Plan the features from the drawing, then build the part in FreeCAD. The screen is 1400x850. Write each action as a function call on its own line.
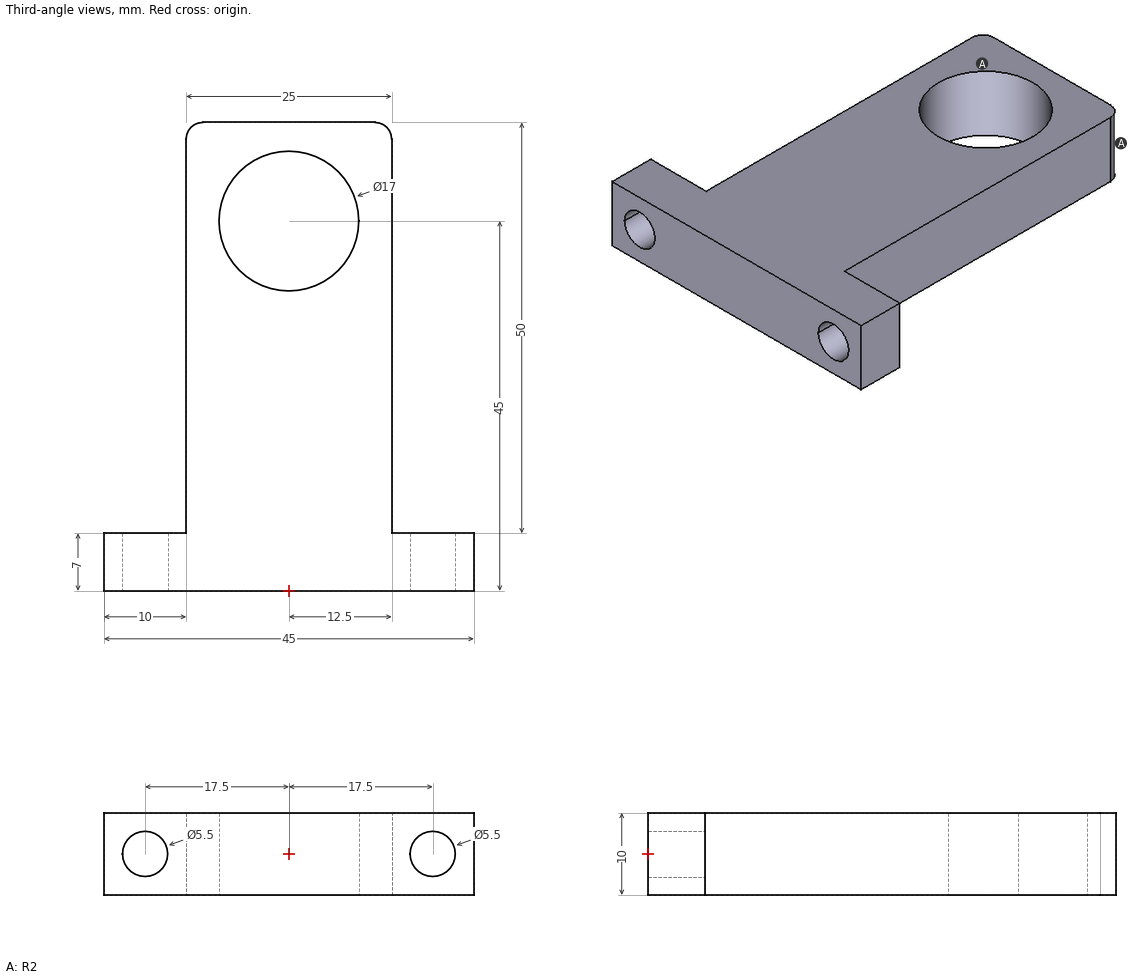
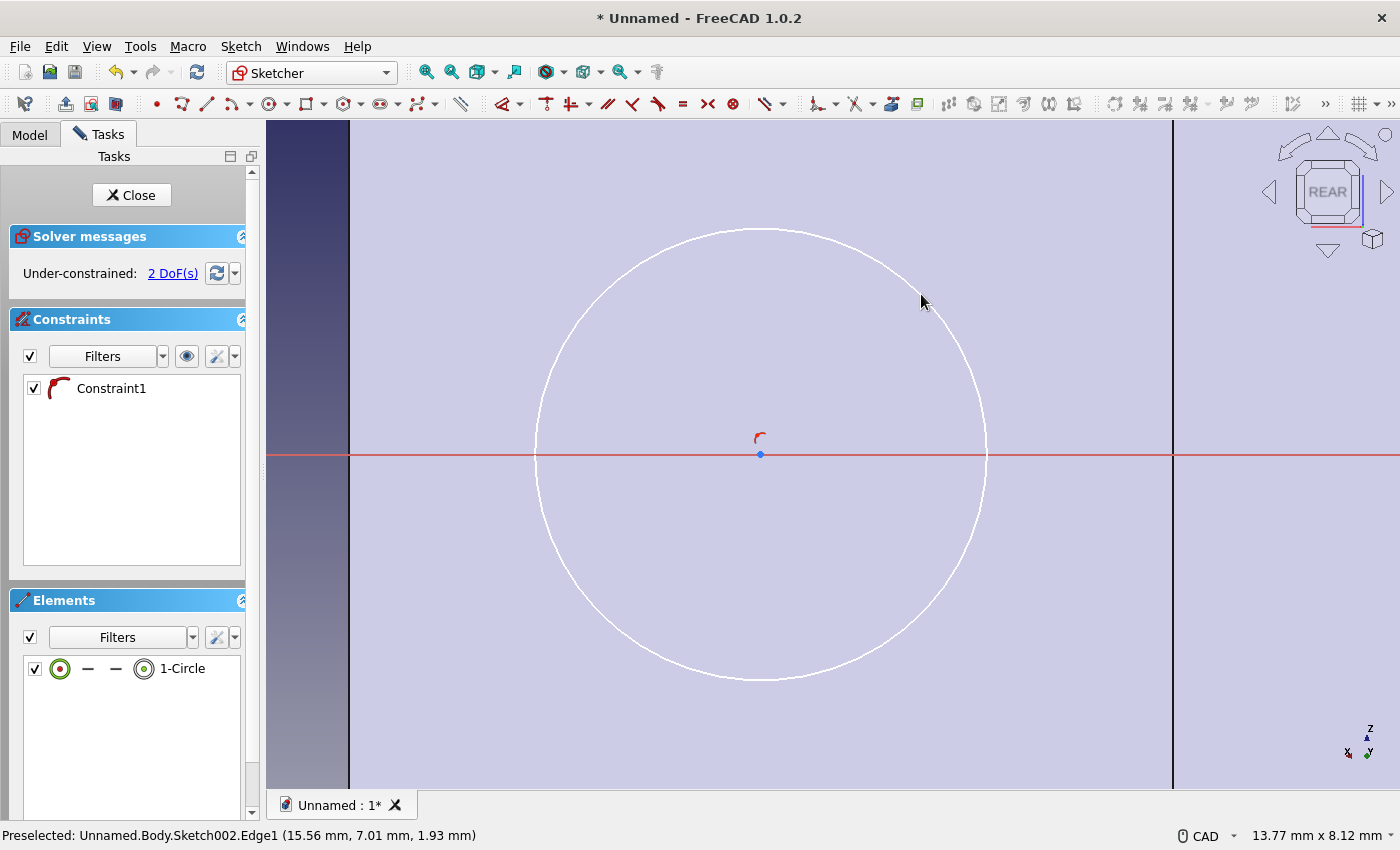
click(502, 104)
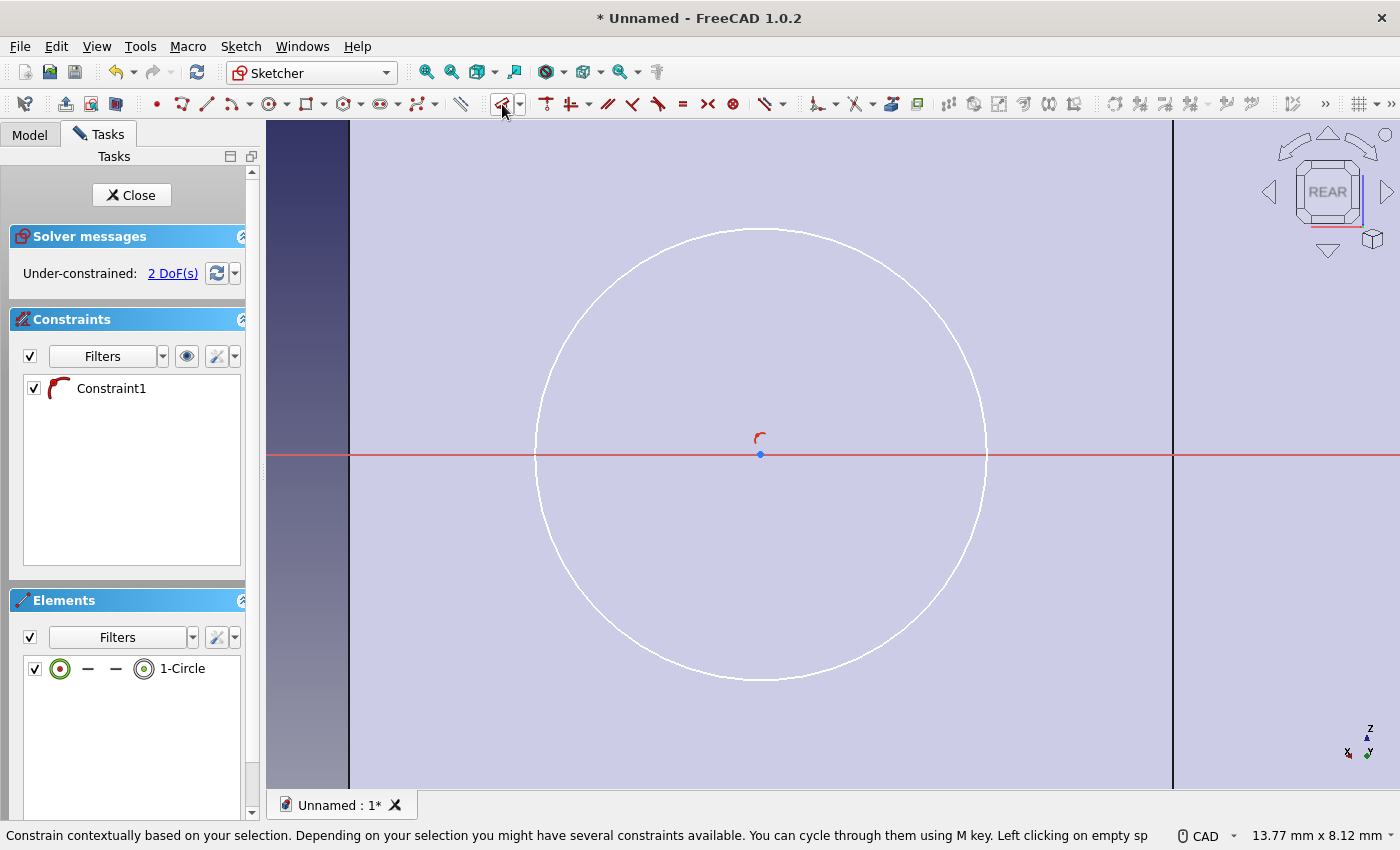
click(920, 294)
click(943, 271)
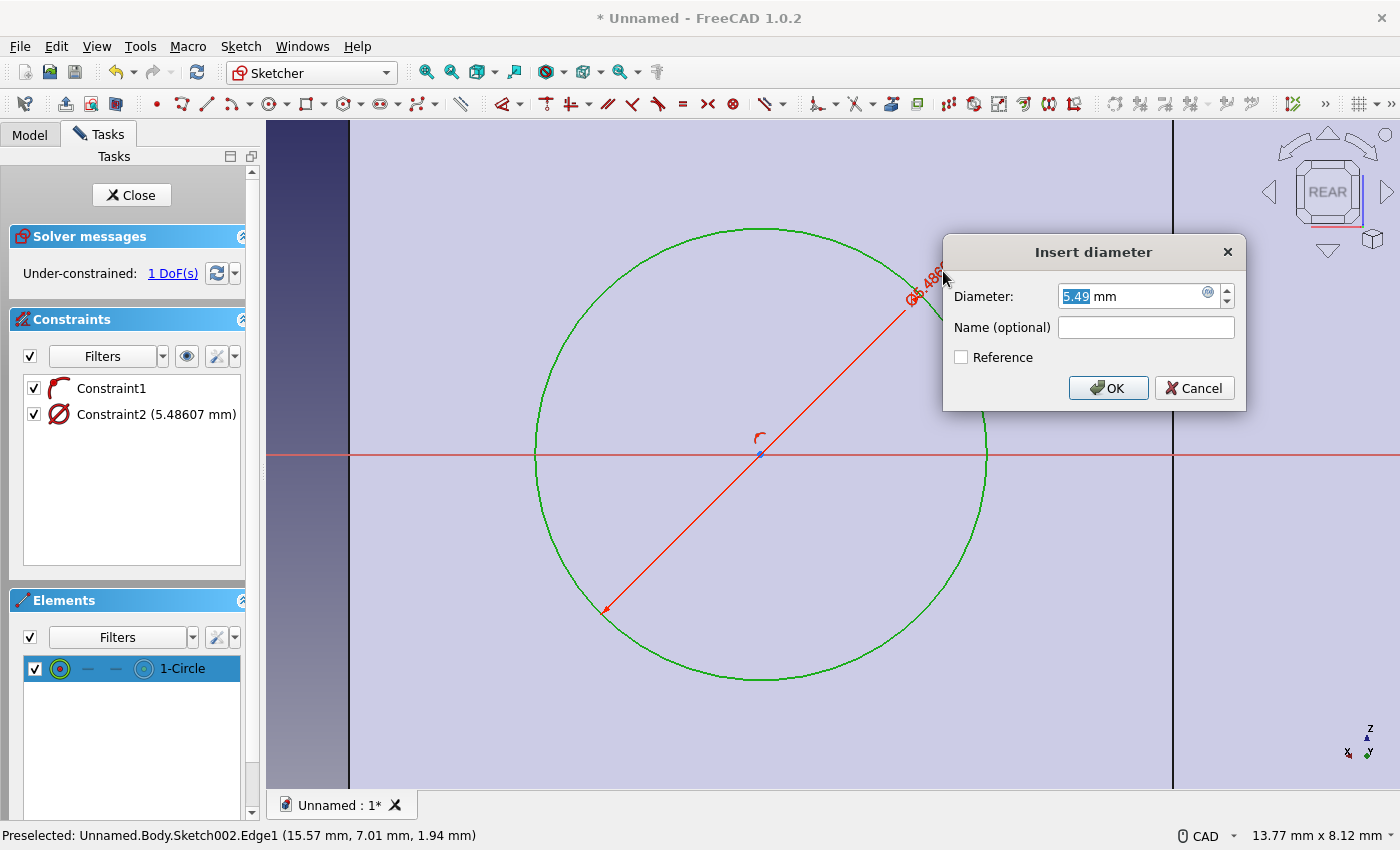
text(5.5)
key(Return)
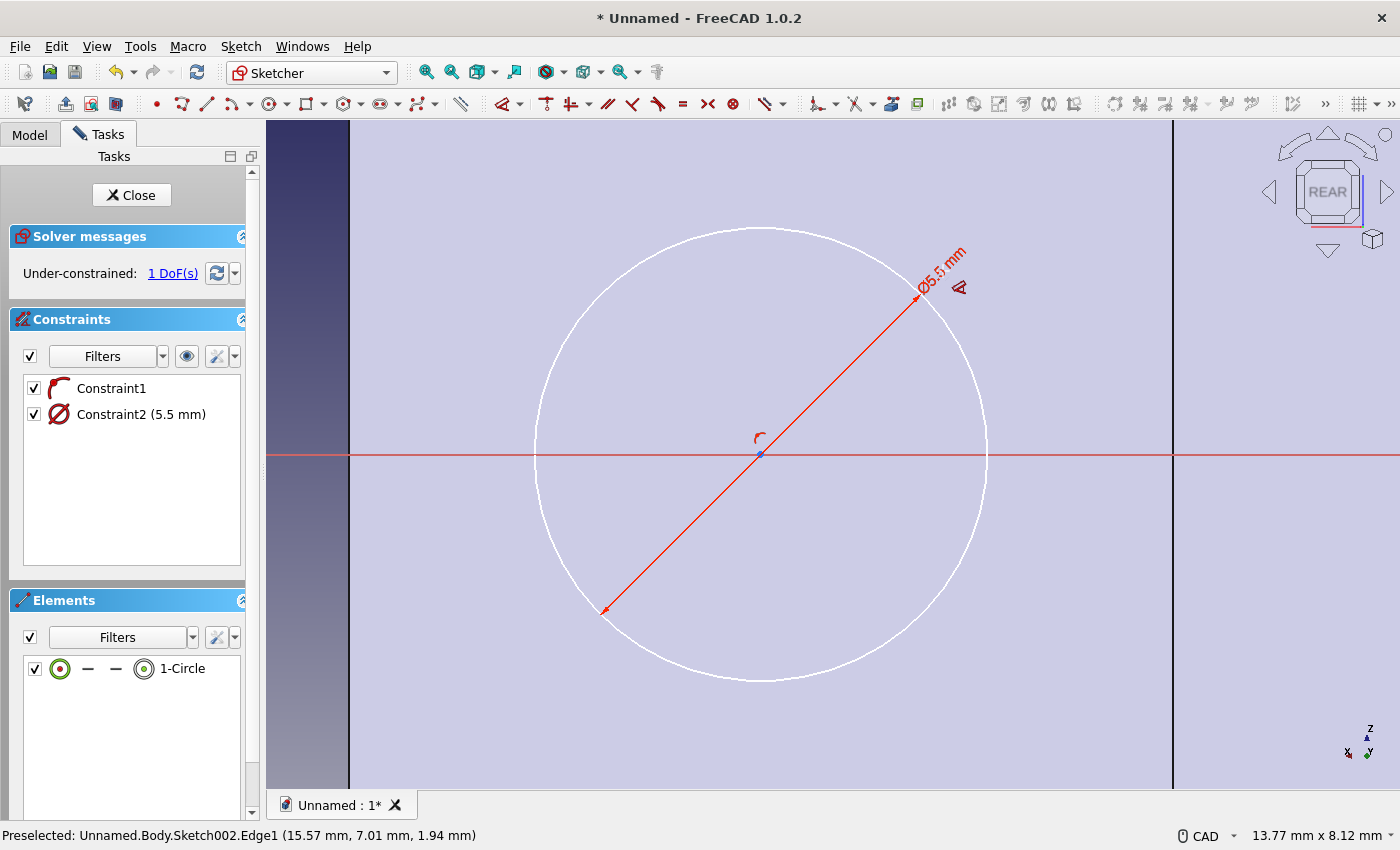
click(761, 454)
click(889, 488)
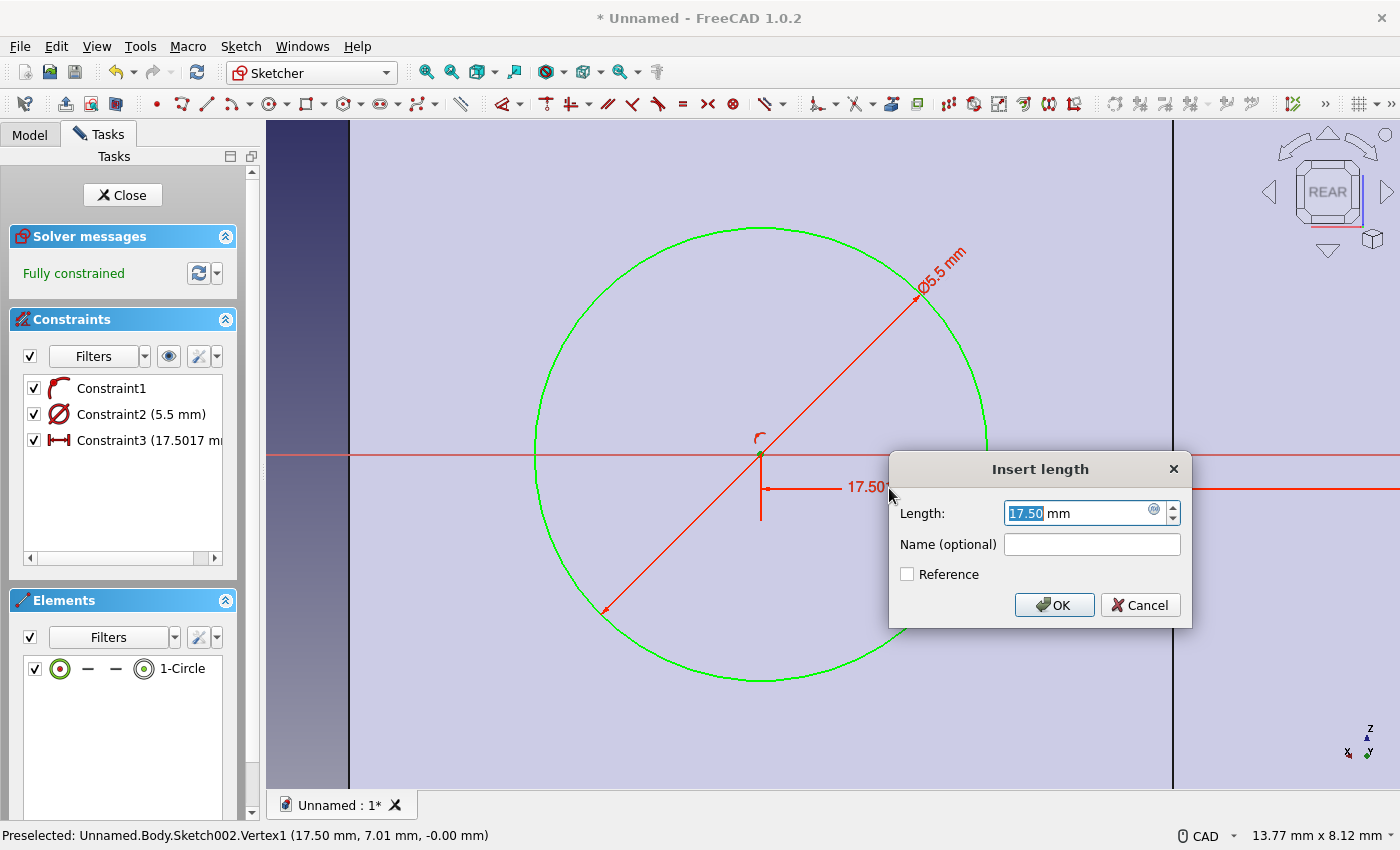
text(17.5)
key(Return)
key(Escape)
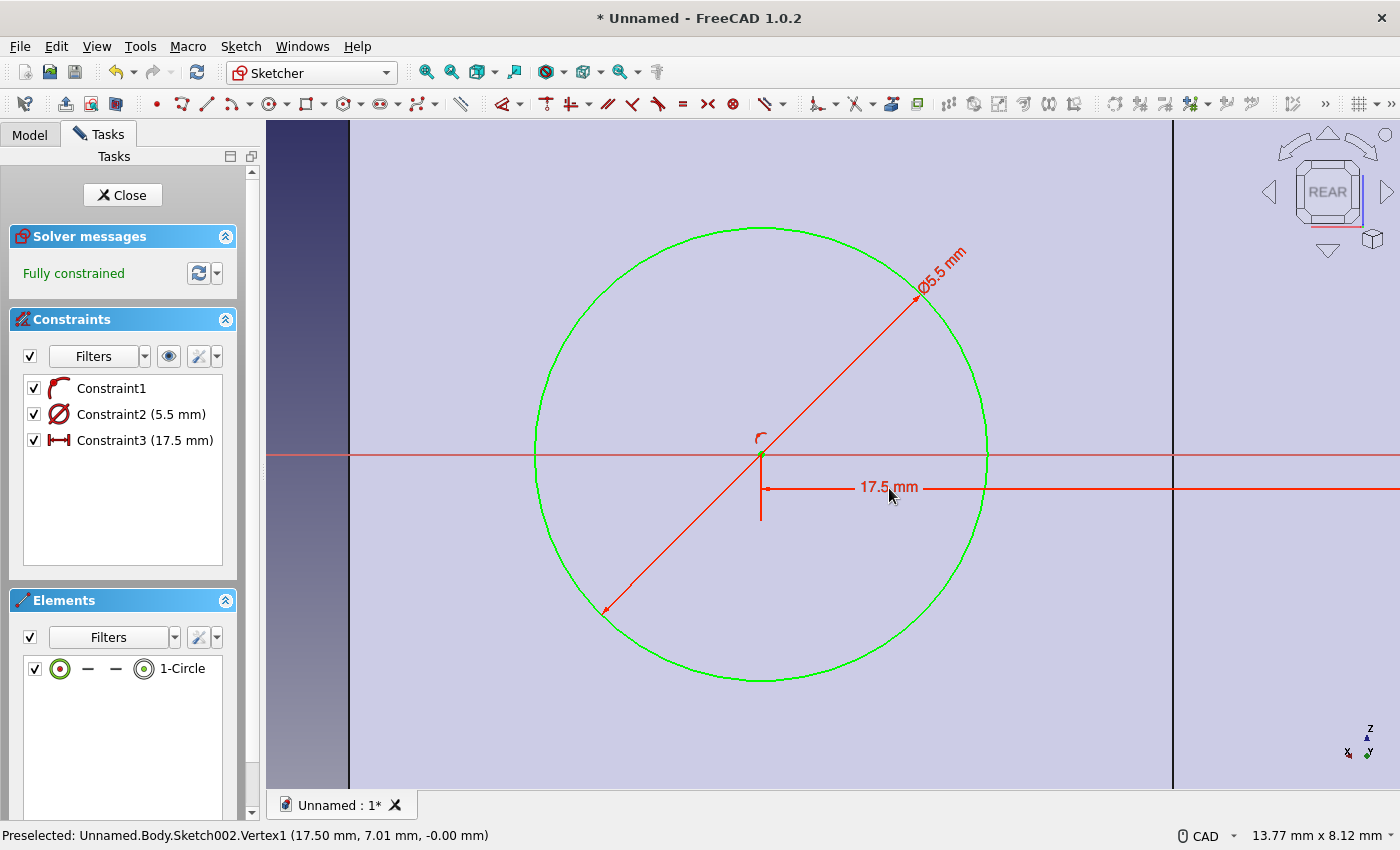
click(123, 195)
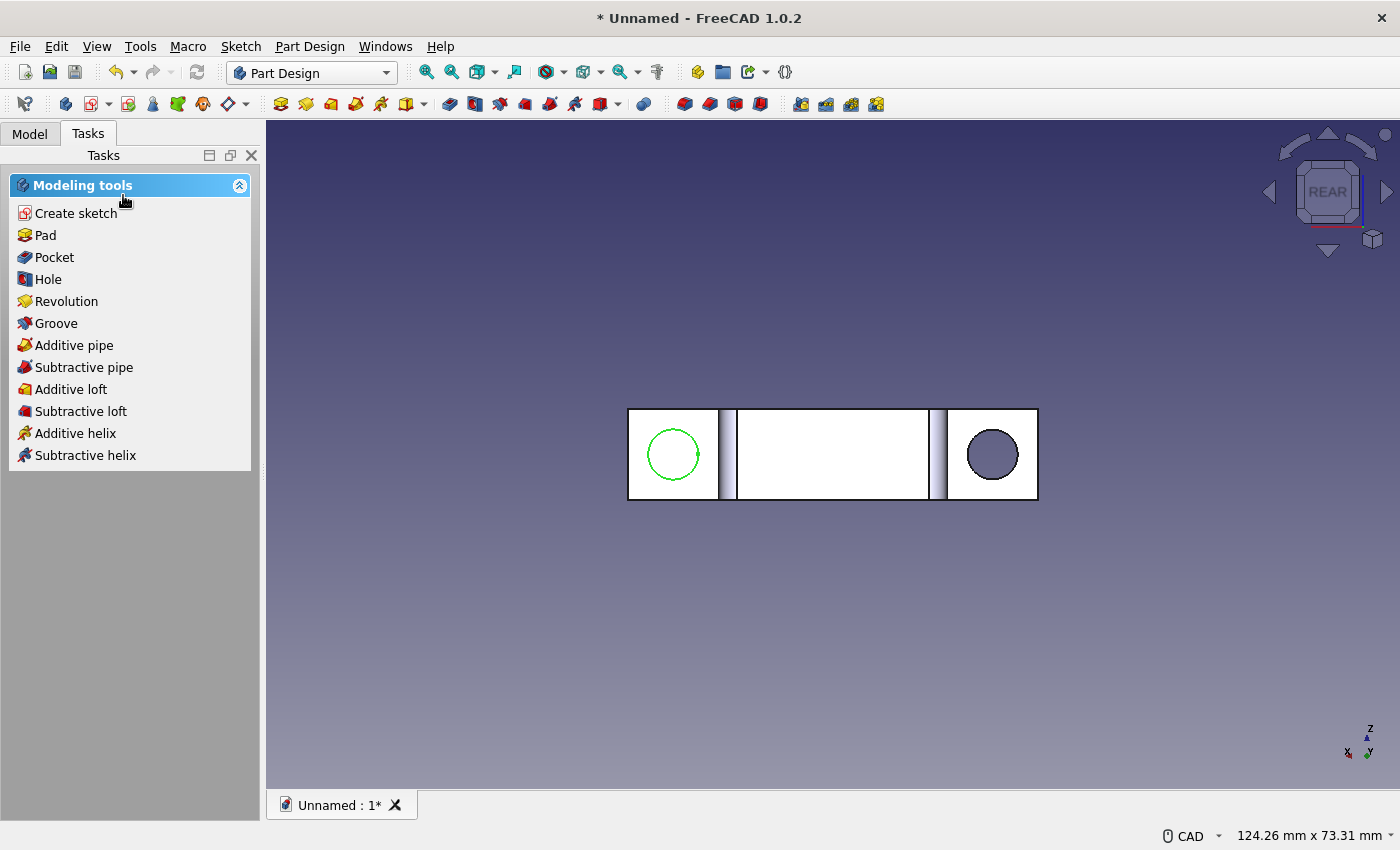
click(450, 104)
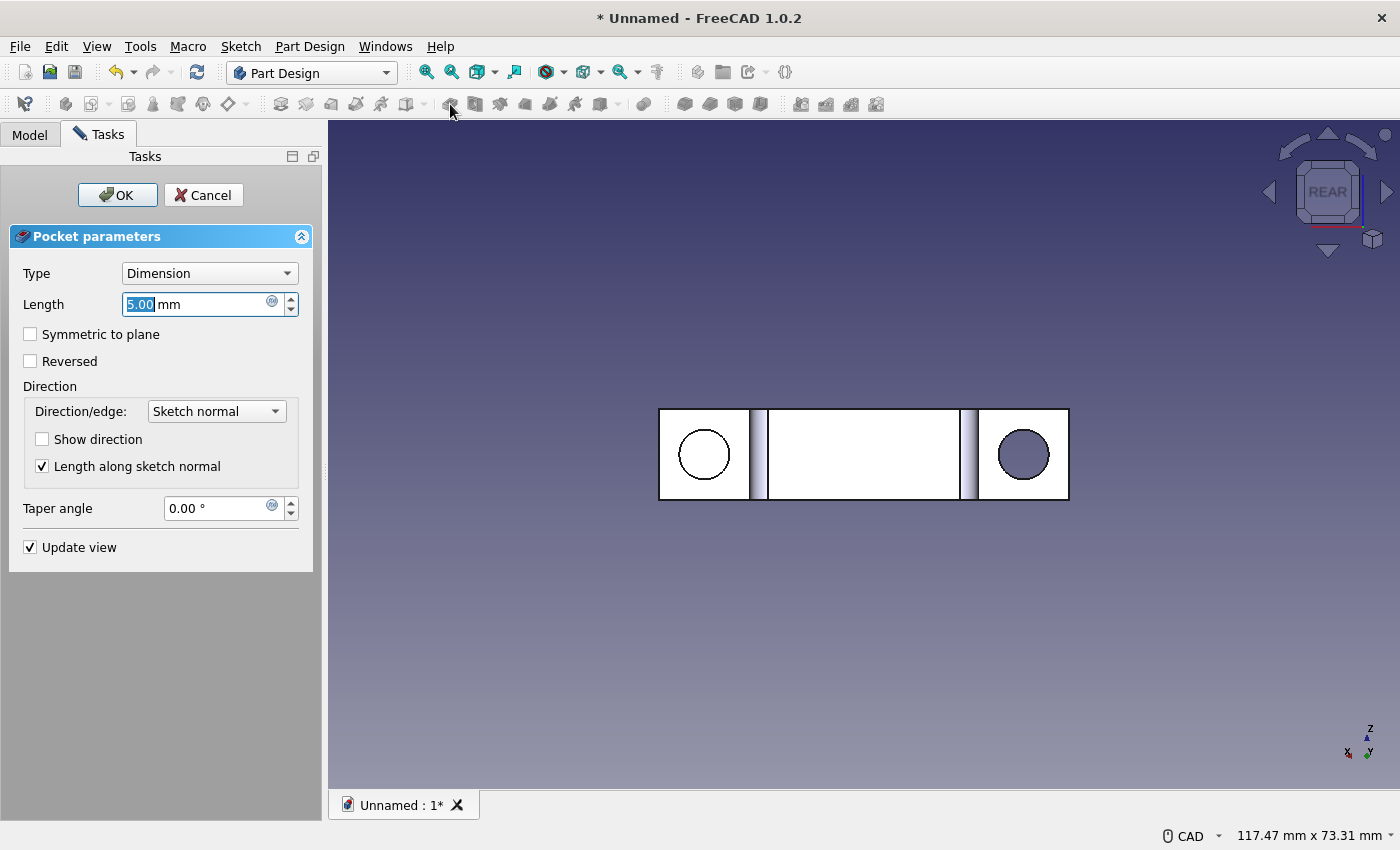
click(210, 274)